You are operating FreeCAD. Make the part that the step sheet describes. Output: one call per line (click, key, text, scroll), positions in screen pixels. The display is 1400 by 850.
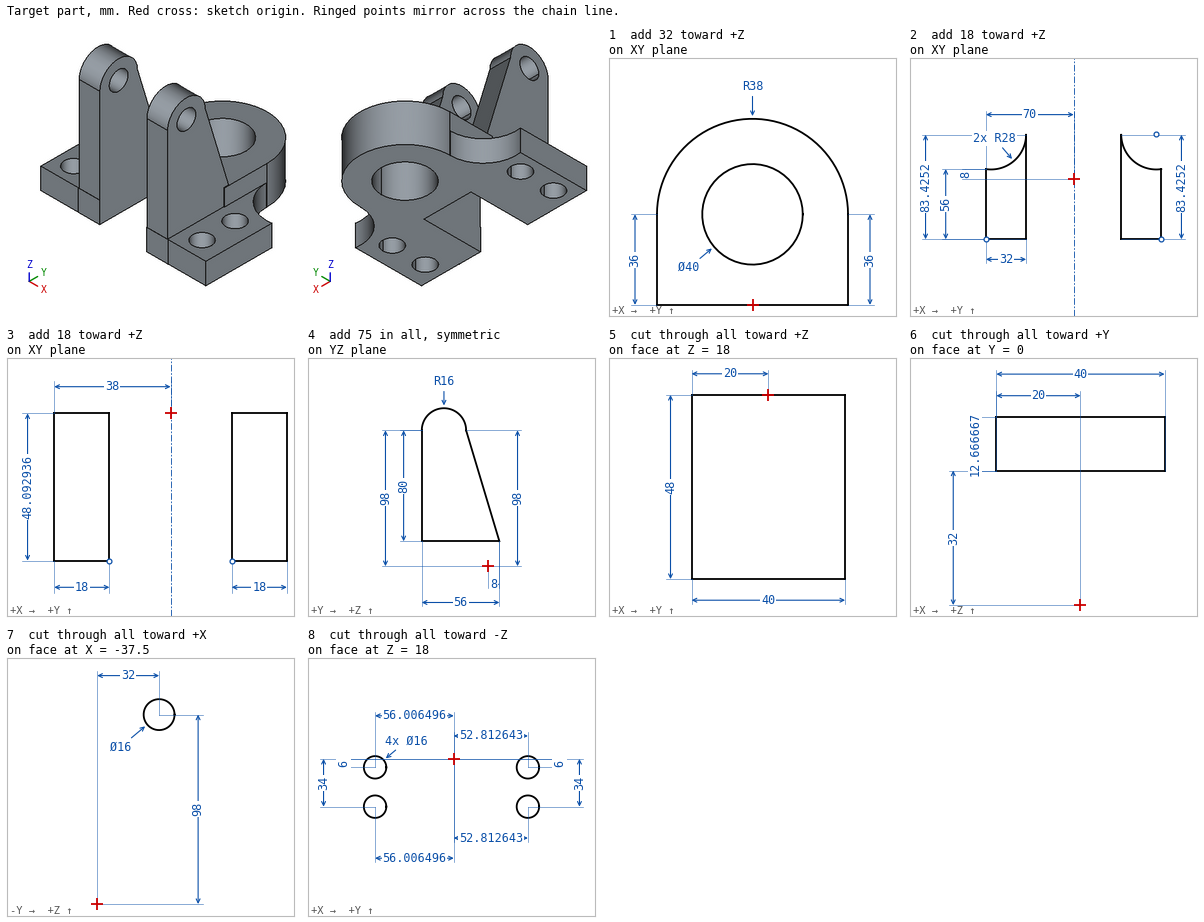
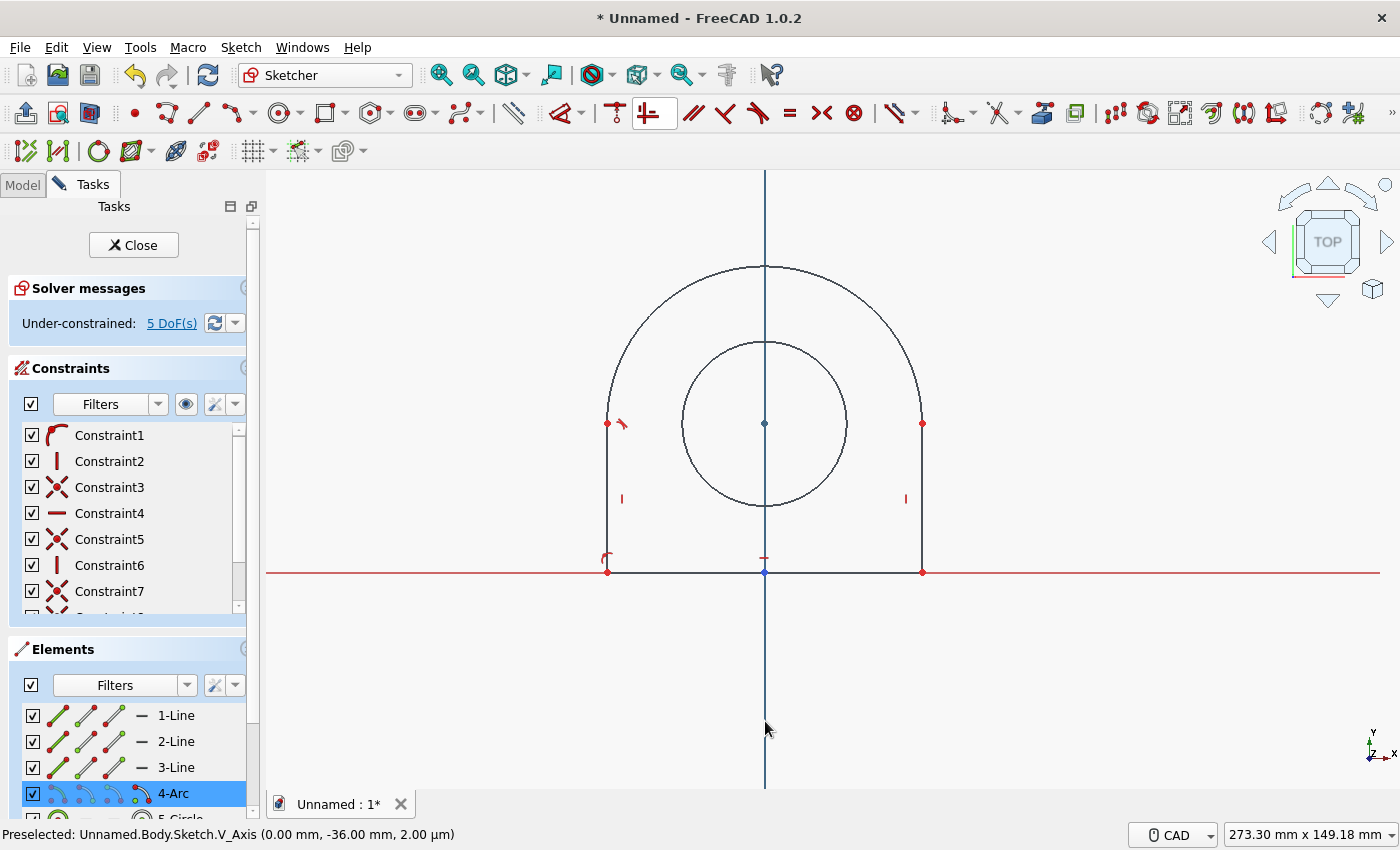
click(616, 114)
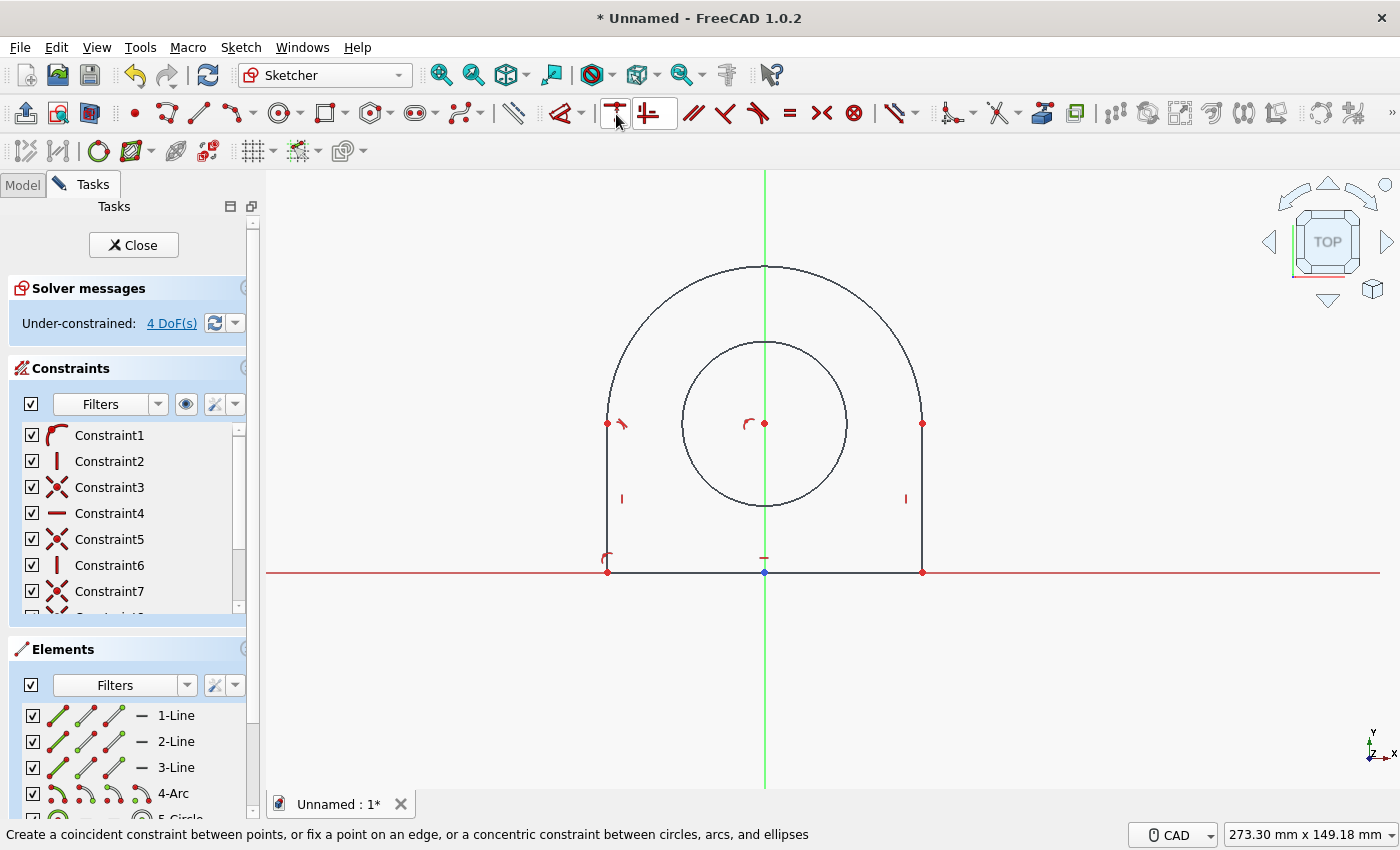
click(560, 114)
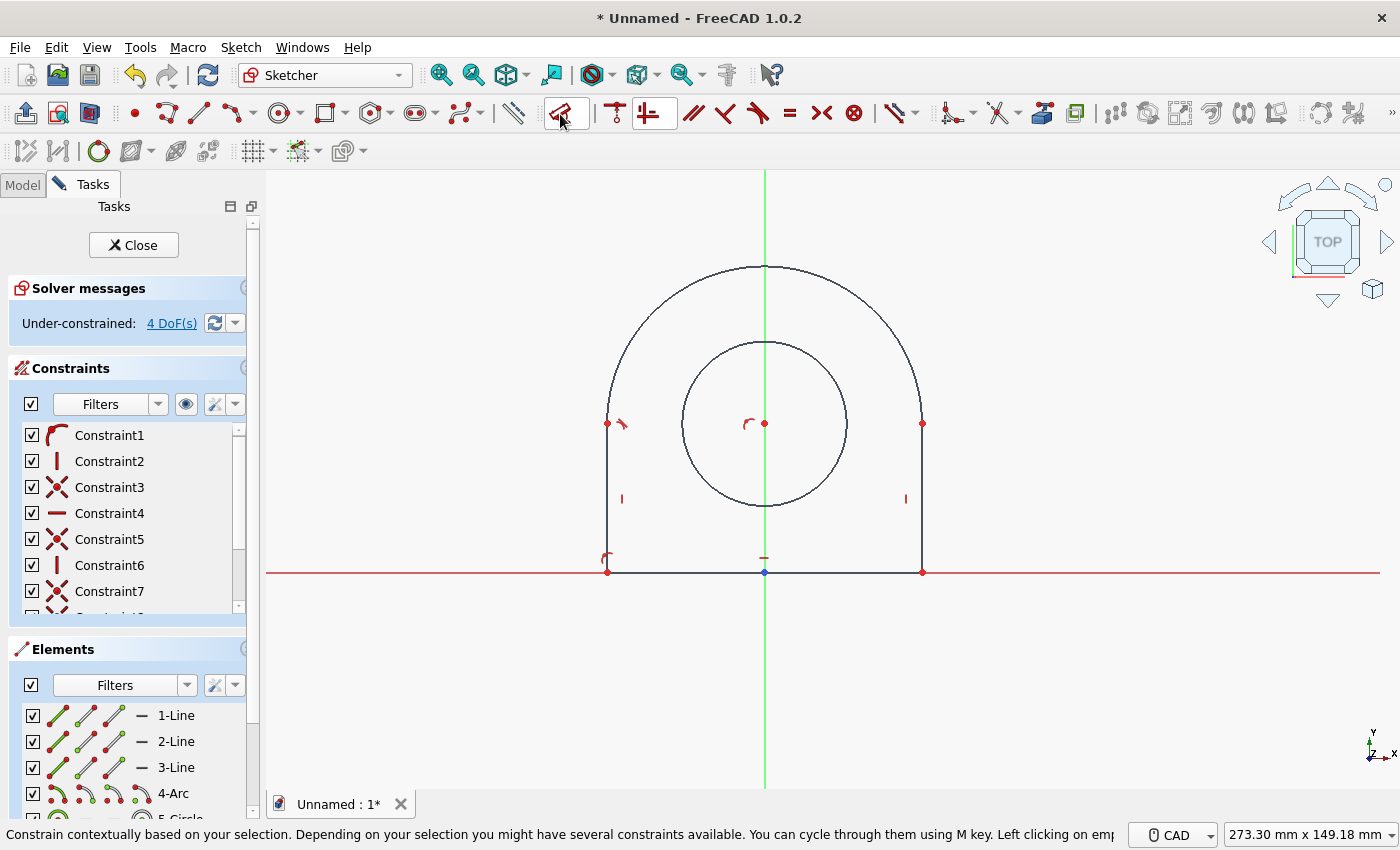
click(857, 297)
click(876, 271)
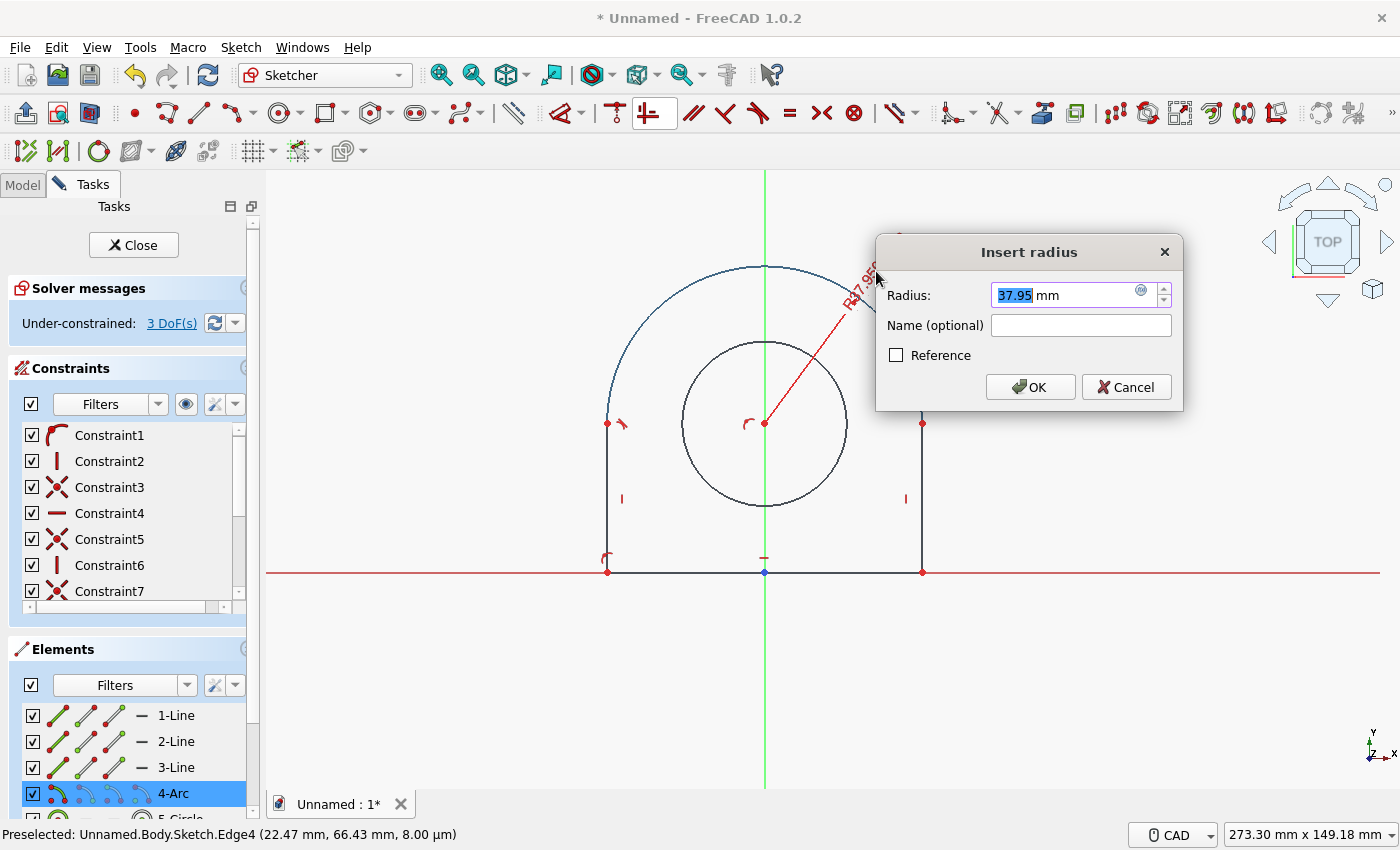
text(38)
key(Return)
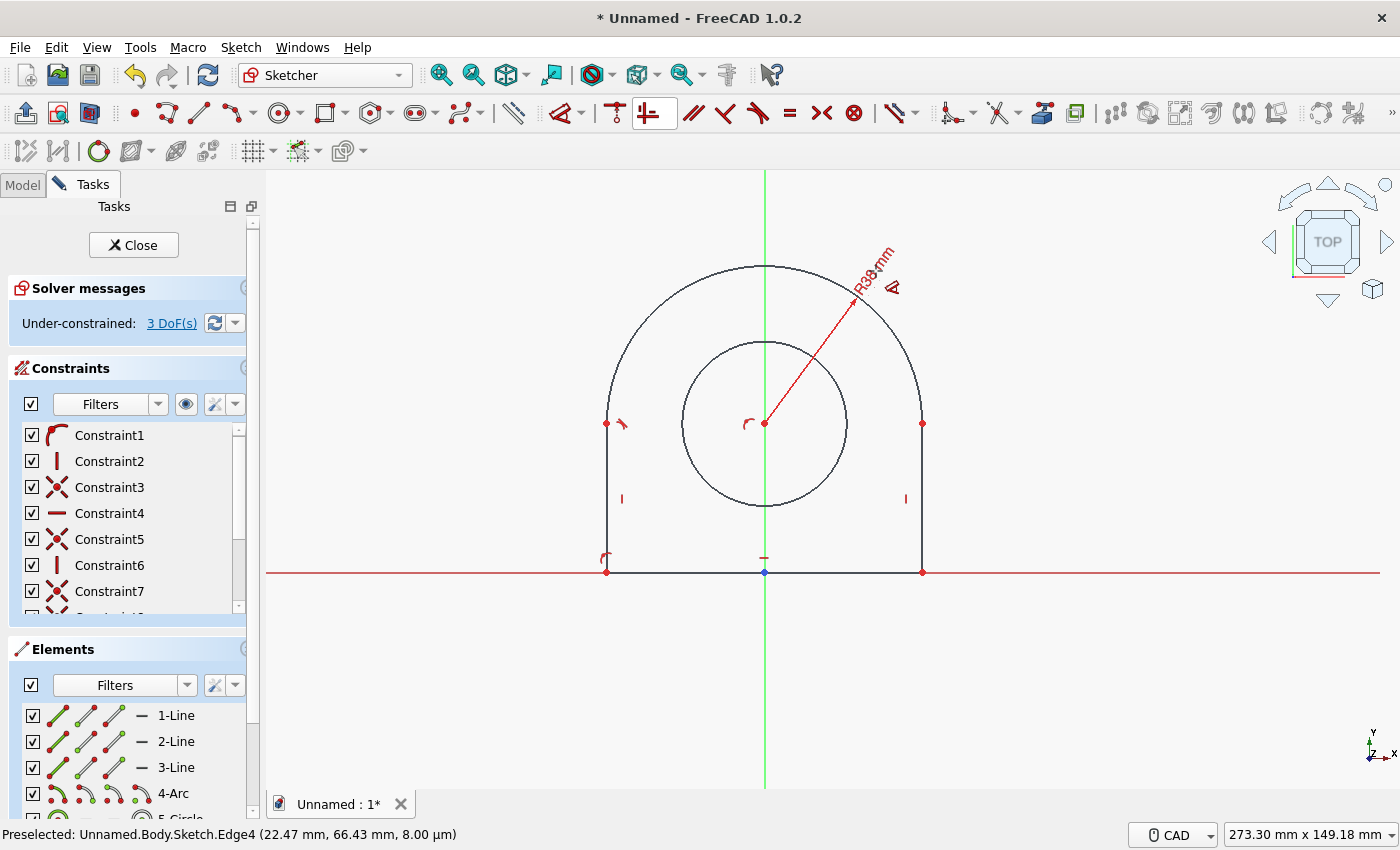
click(823, 365)
click(846, 342)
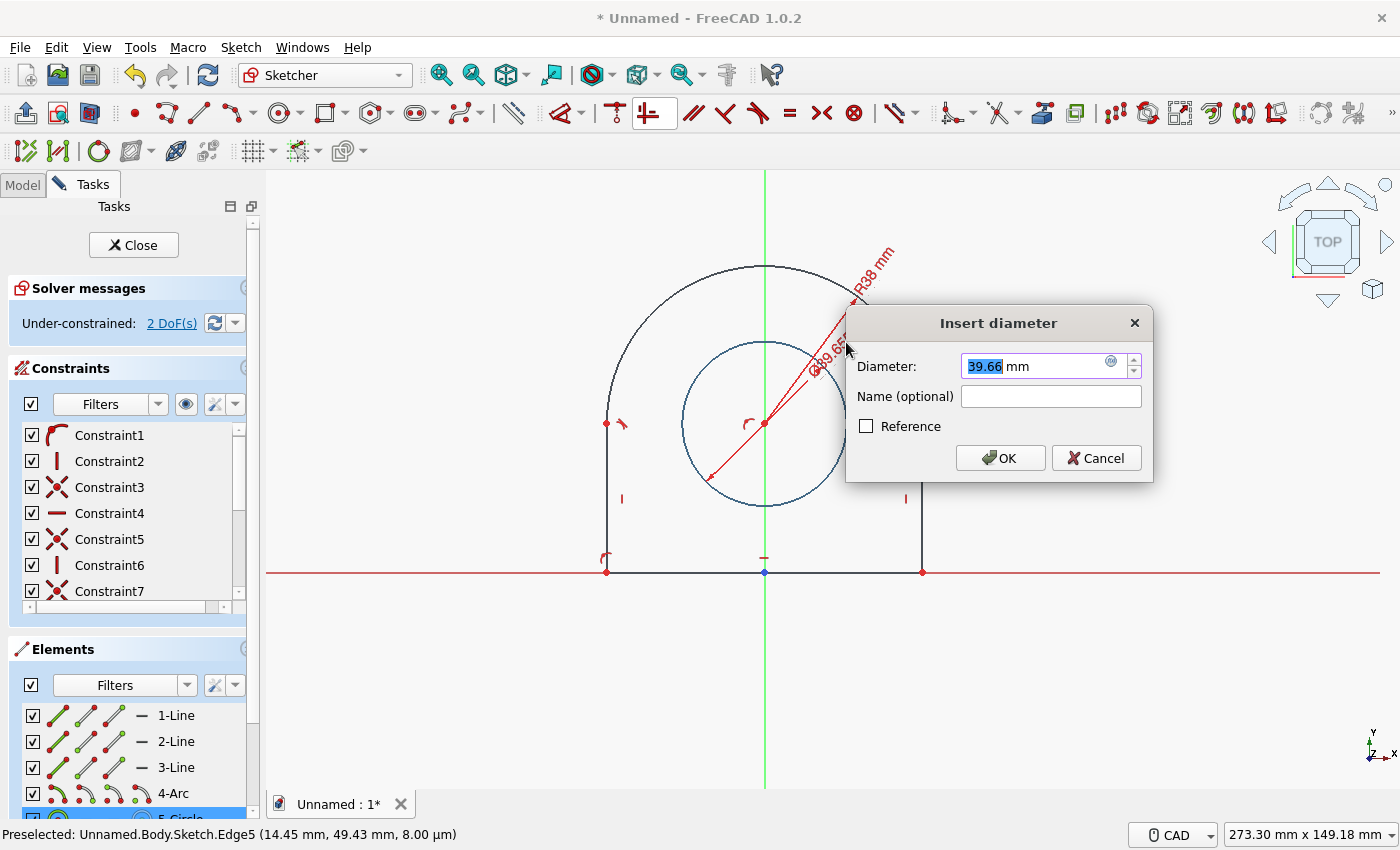
text(40)
key(Return)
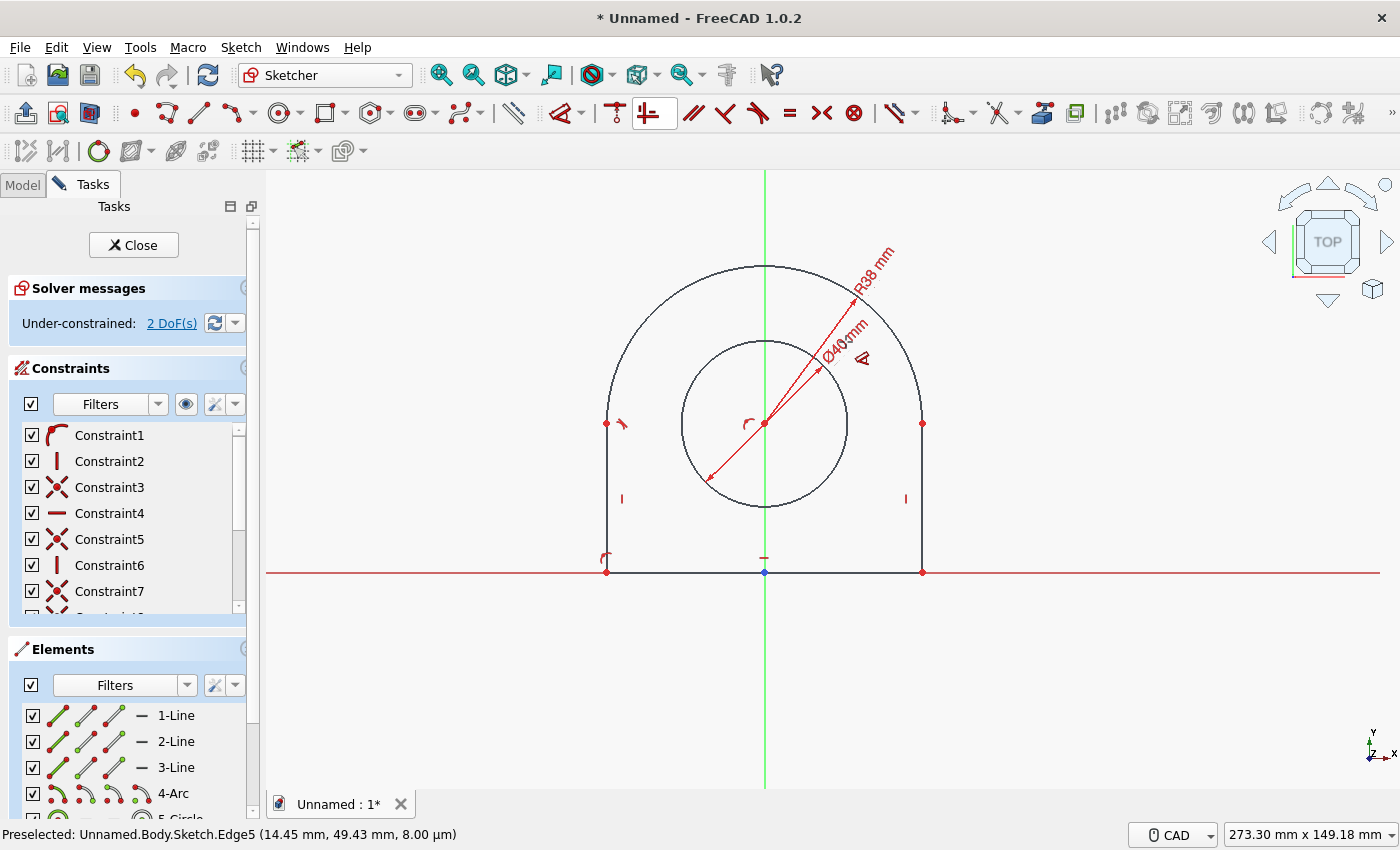
click(607, 468)
click(573, 498)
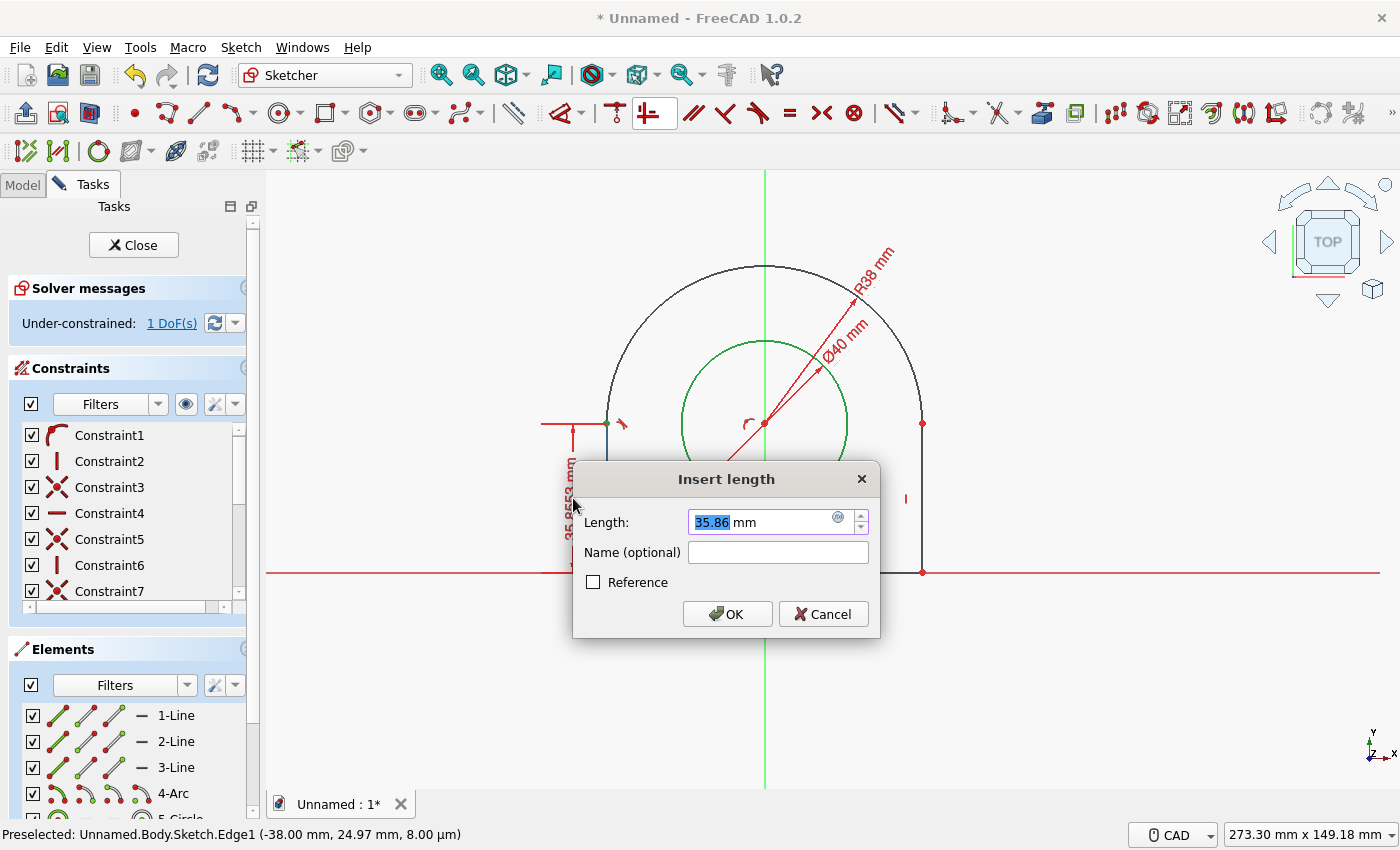
text(36)
key(Return)